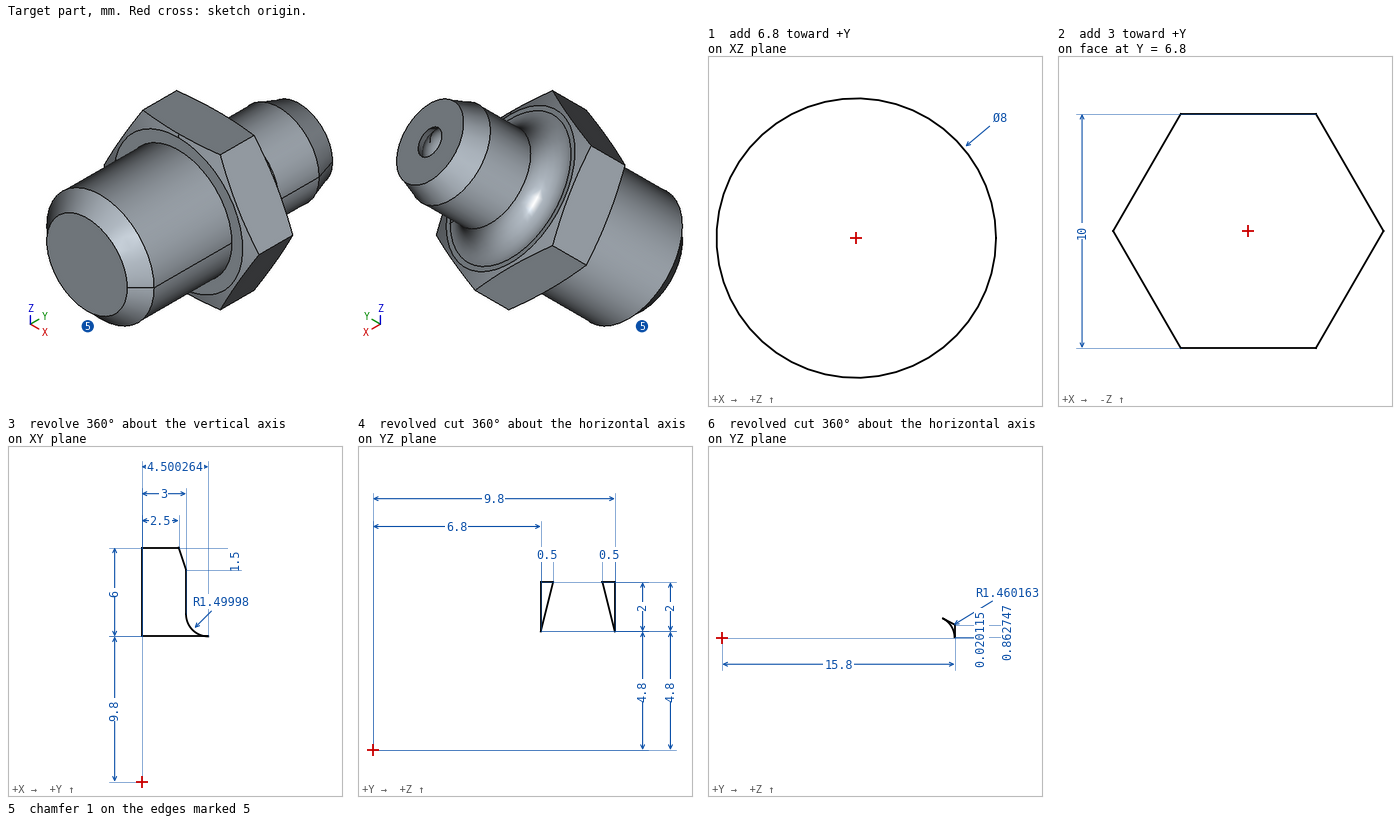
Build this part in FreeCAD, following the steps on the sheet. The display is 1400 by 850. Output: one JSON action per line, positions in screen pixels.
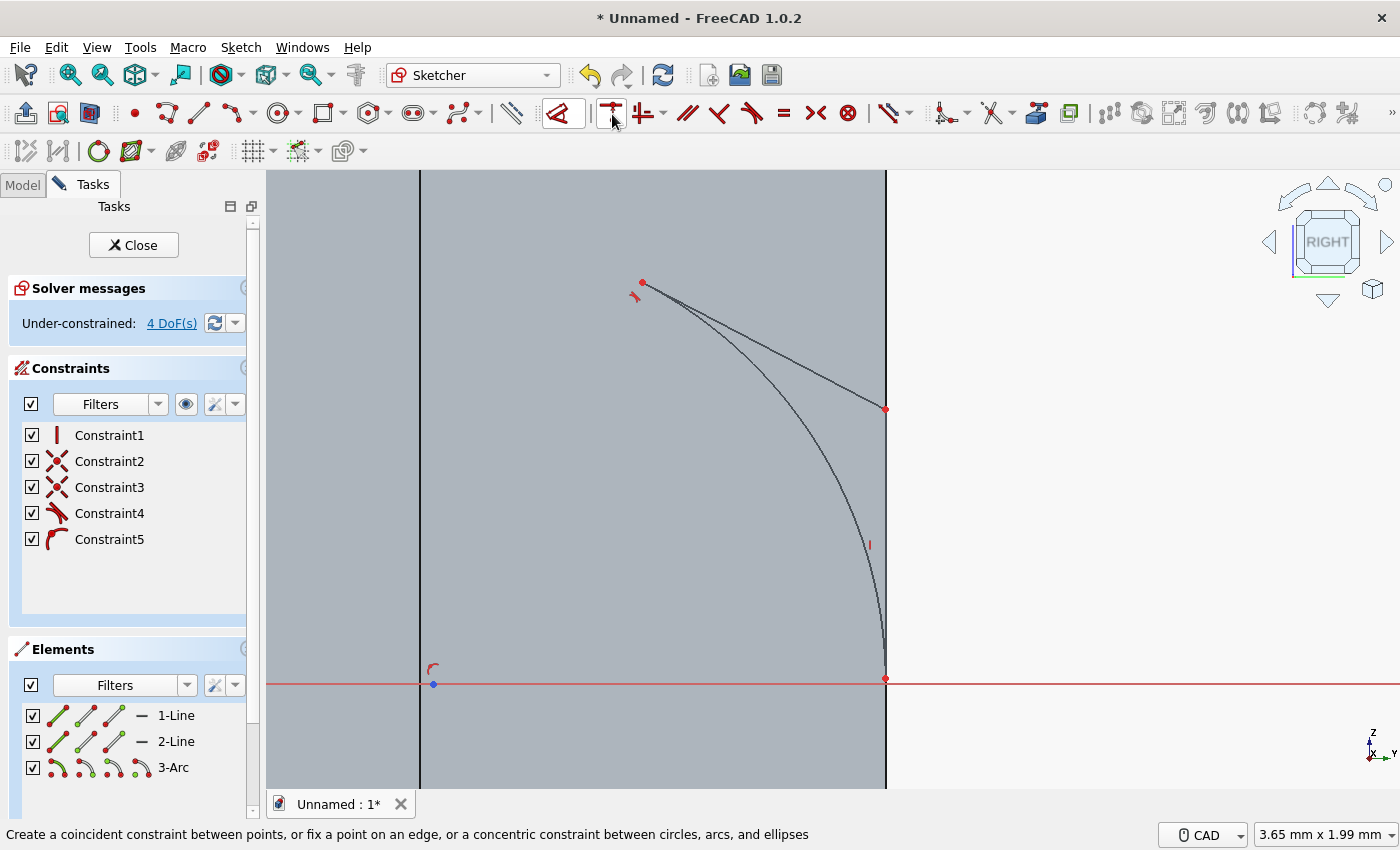
{"action": "left_click", "coordinate": [861, 535]}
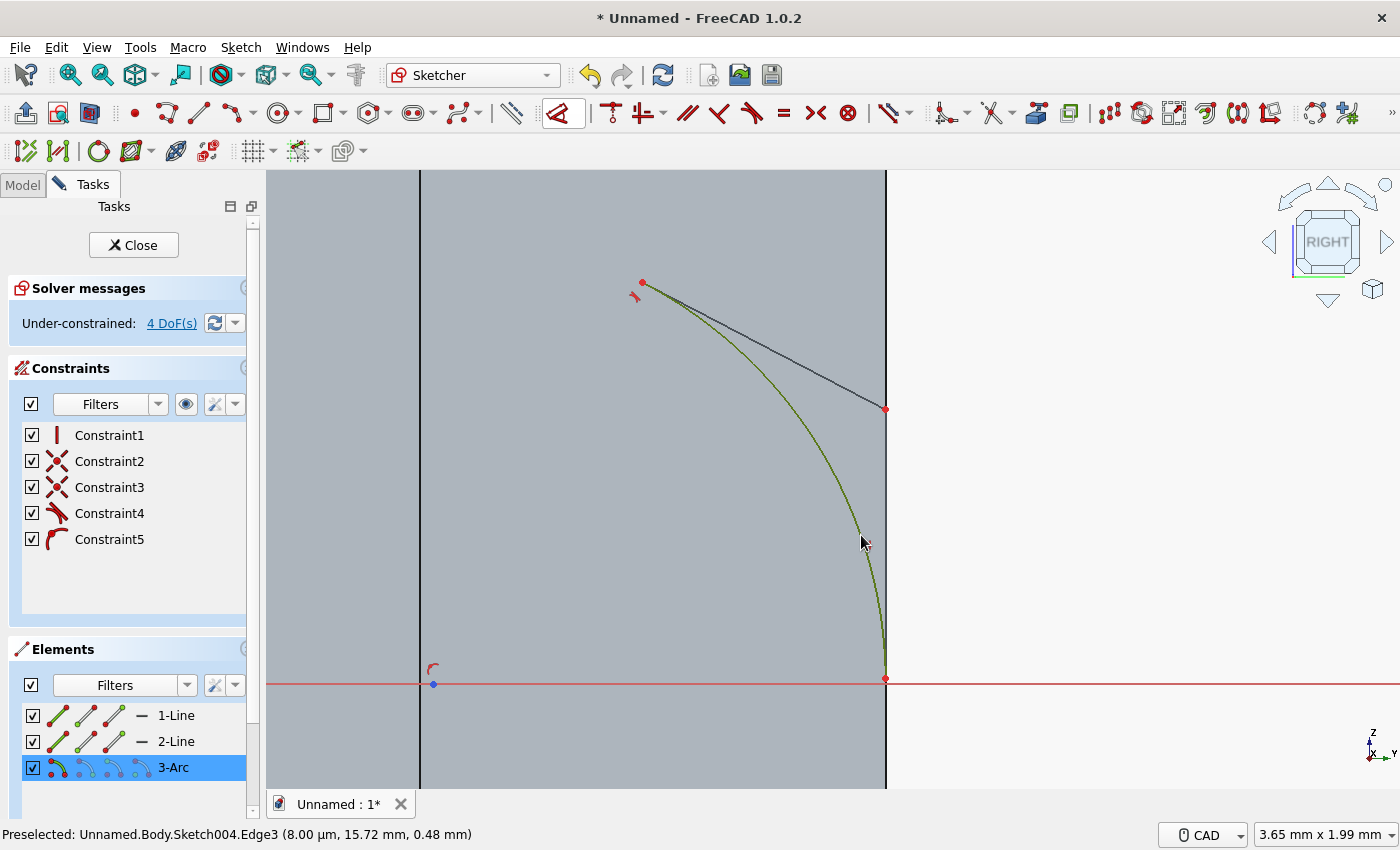
{"action": "key", "text": "k r"}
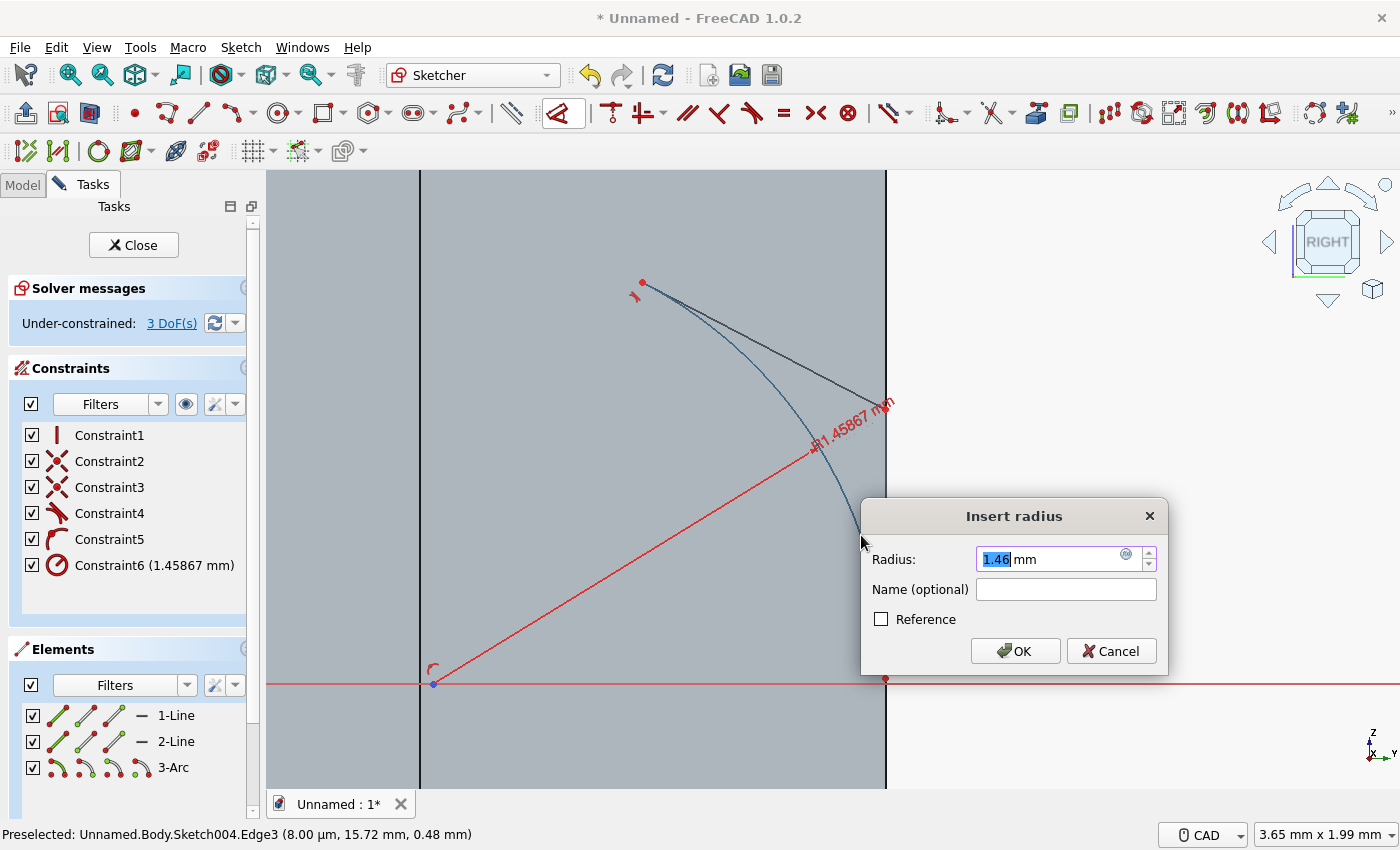
{"action": "type", "text": "1.460163"}
{"action": "key", "text": "Return"}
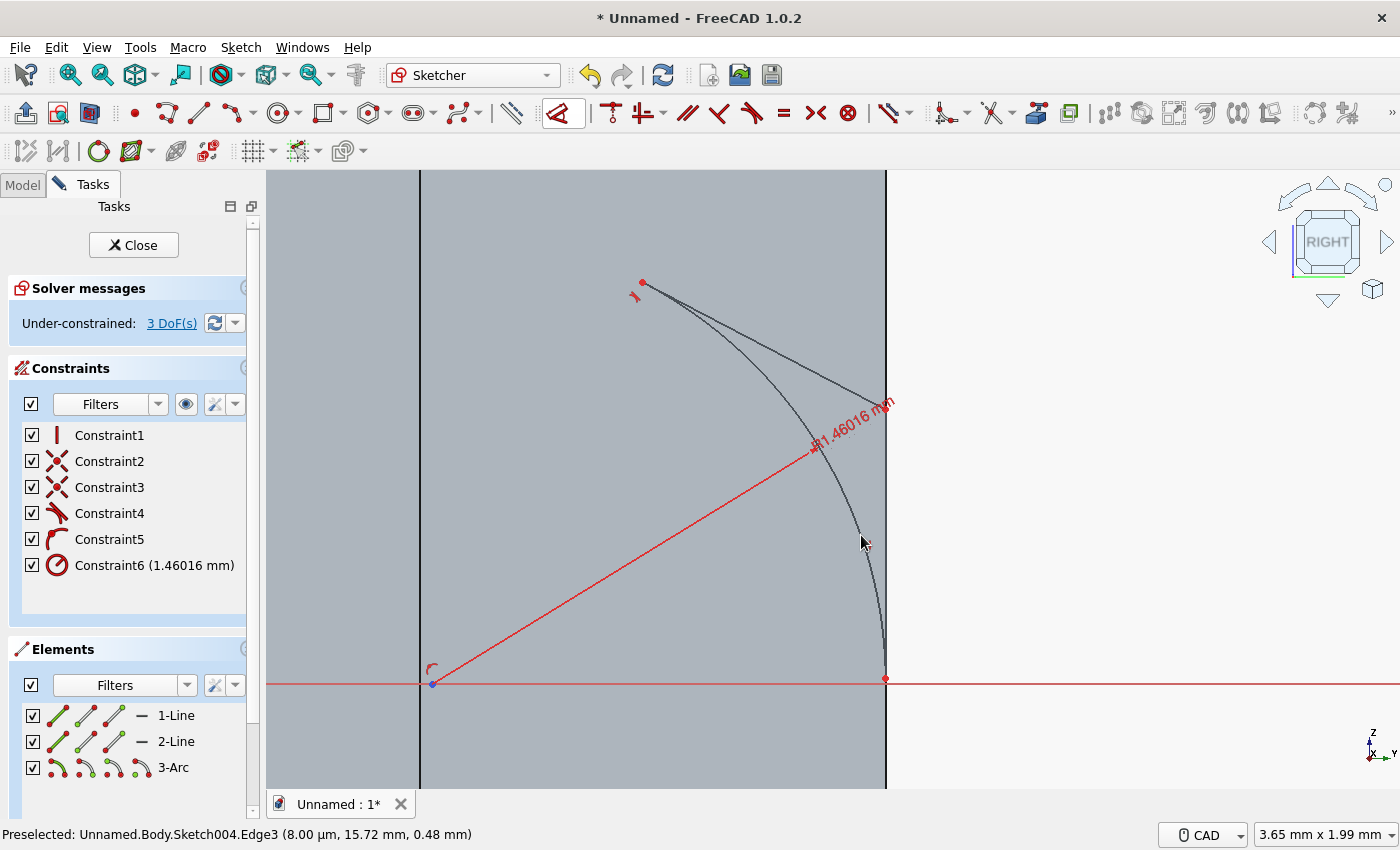
{"action": "left_click", "coordinate": [886, 678]}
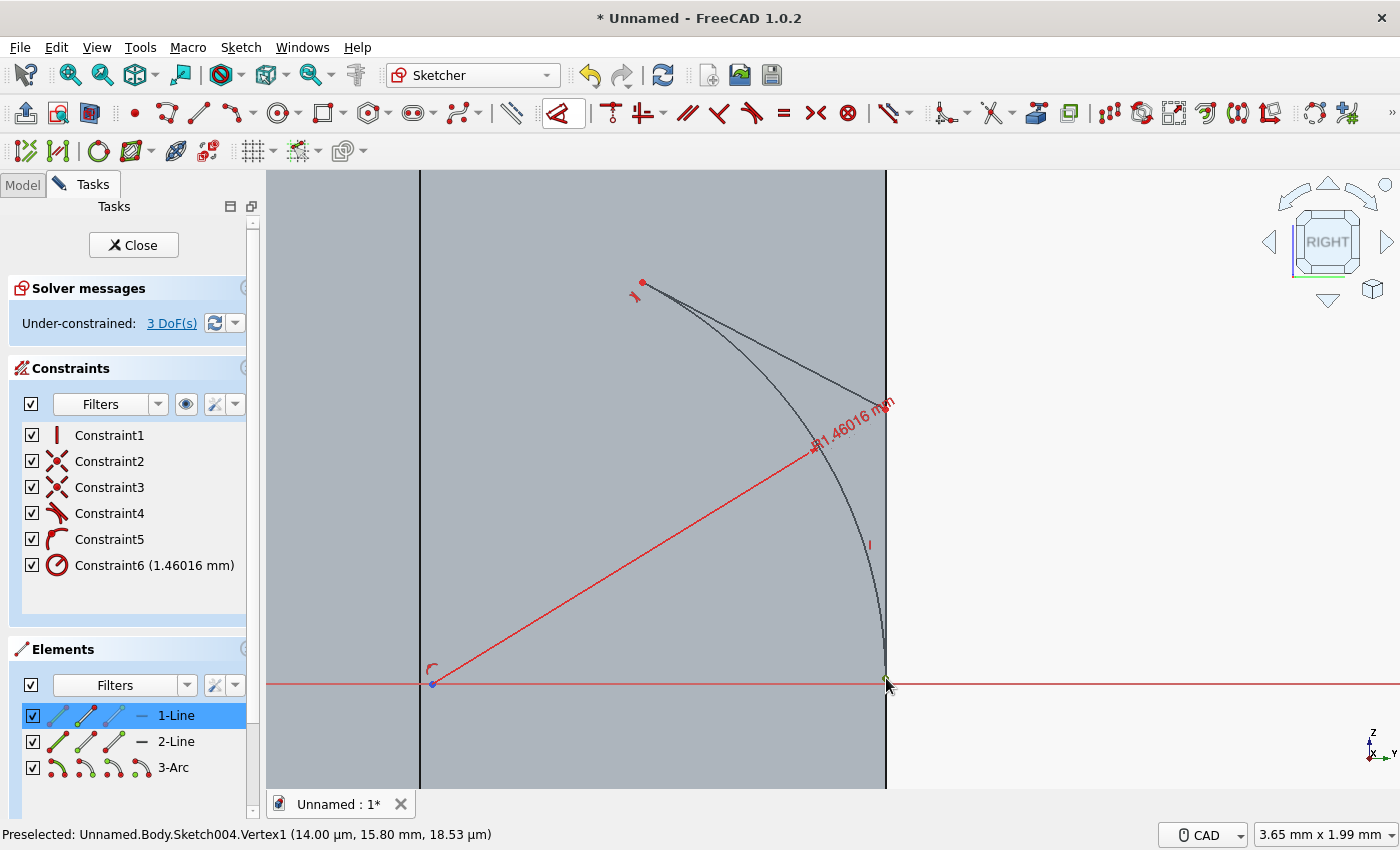
{"action": "key", "text": "l"}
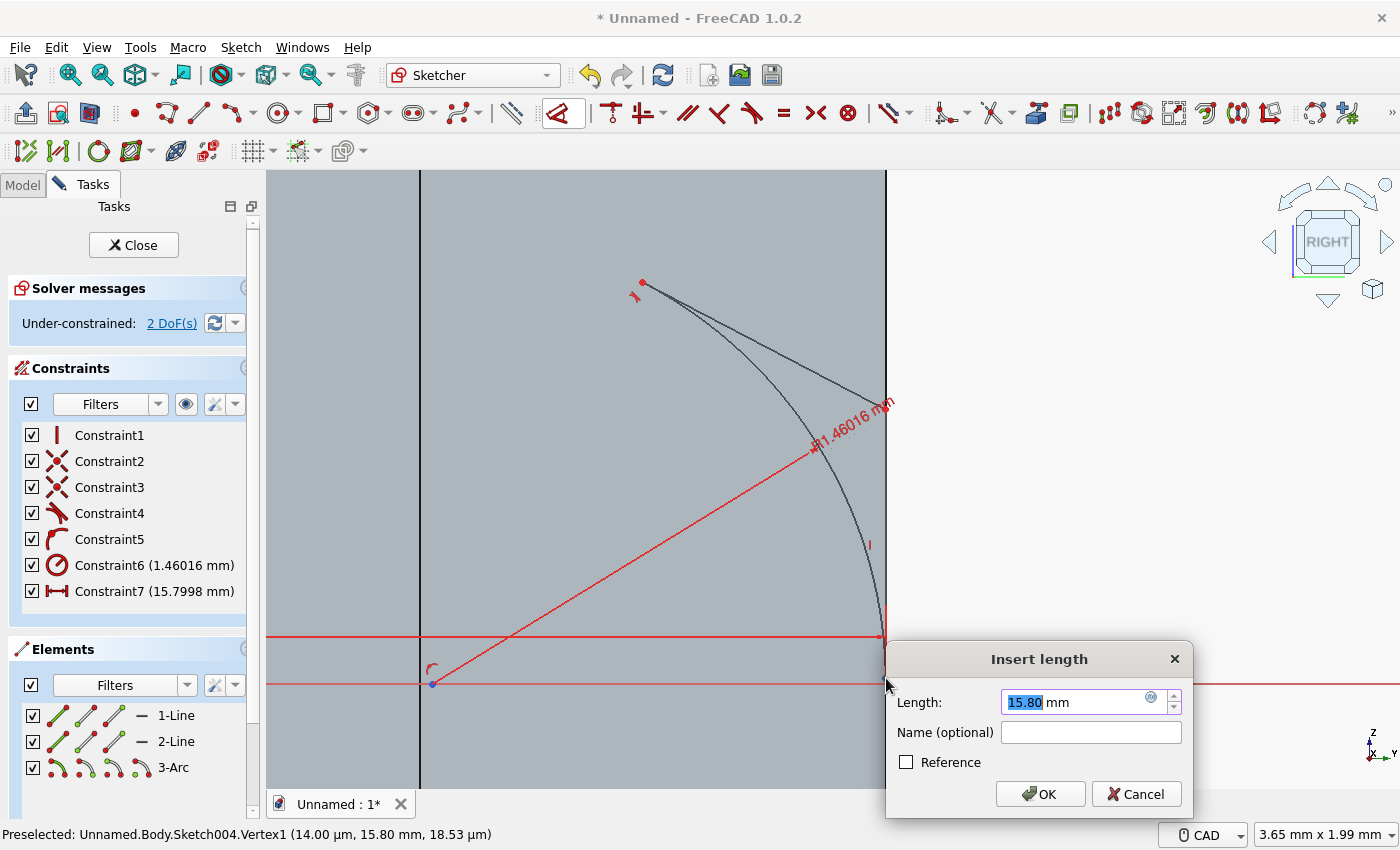
{"action": "type", "text": "15.8"}
{"action": "key", "text": "Return"}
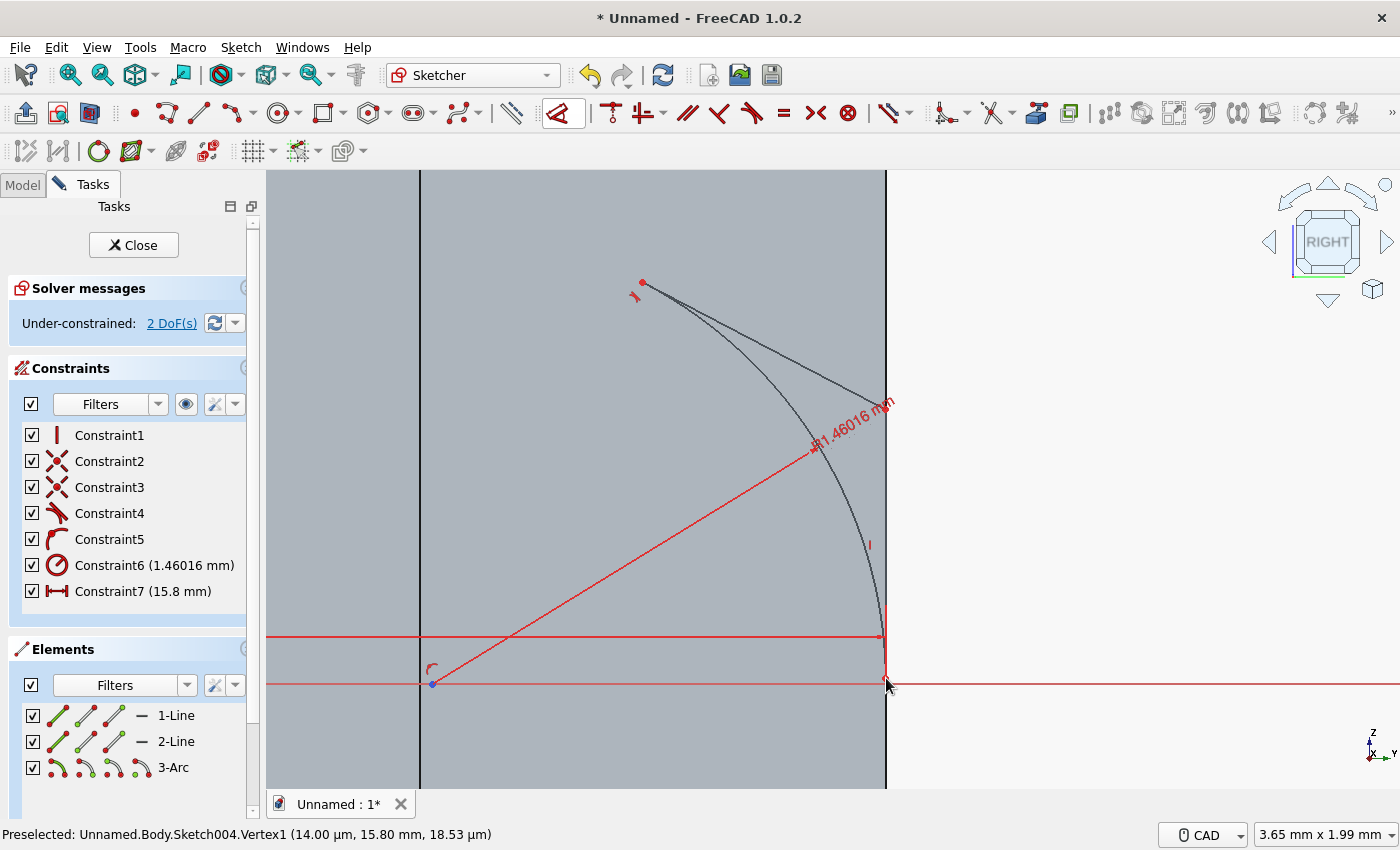
{"action": "left_click", "coordinate": [886, 490]}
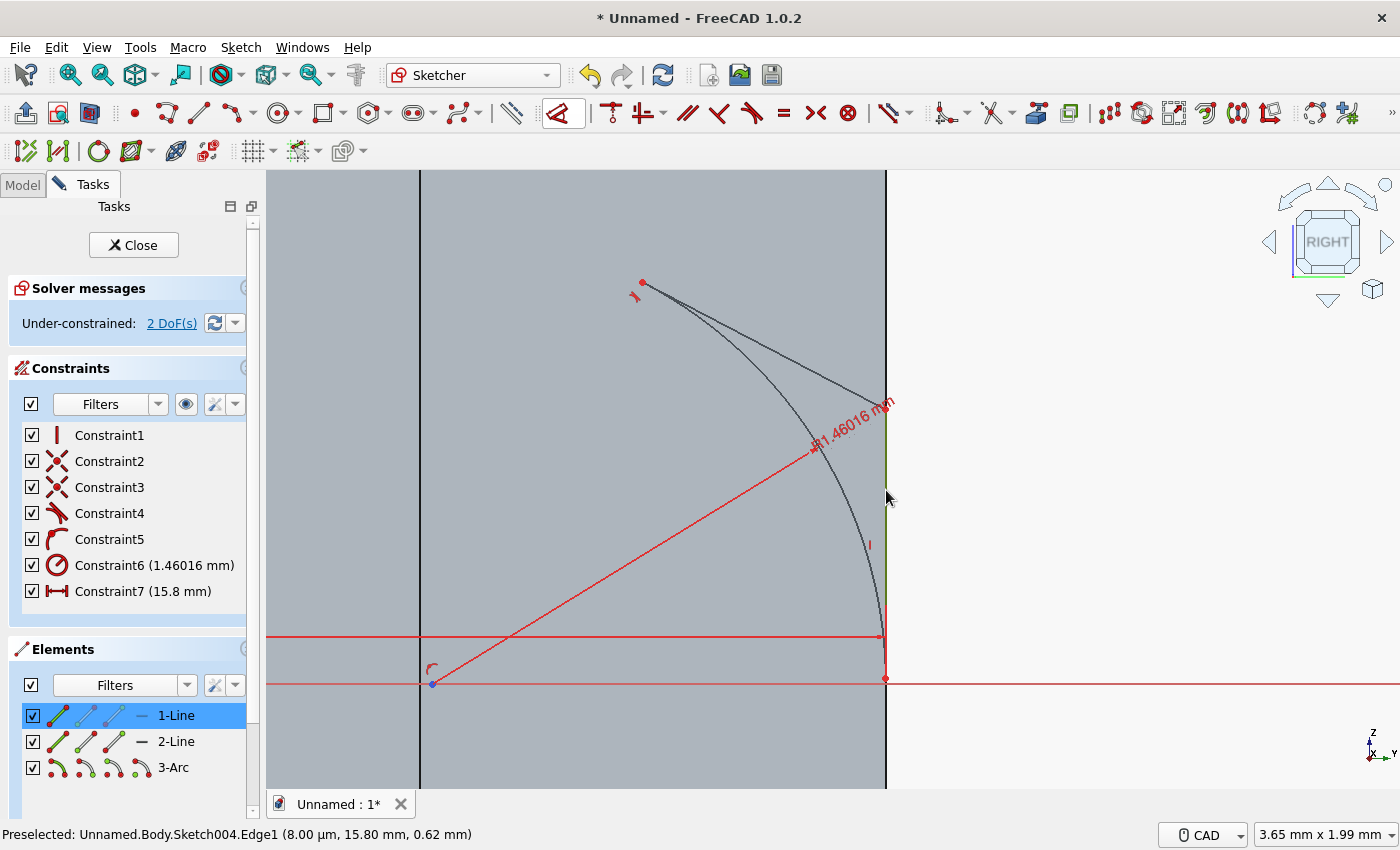
{"action": "key", "text": "i"}